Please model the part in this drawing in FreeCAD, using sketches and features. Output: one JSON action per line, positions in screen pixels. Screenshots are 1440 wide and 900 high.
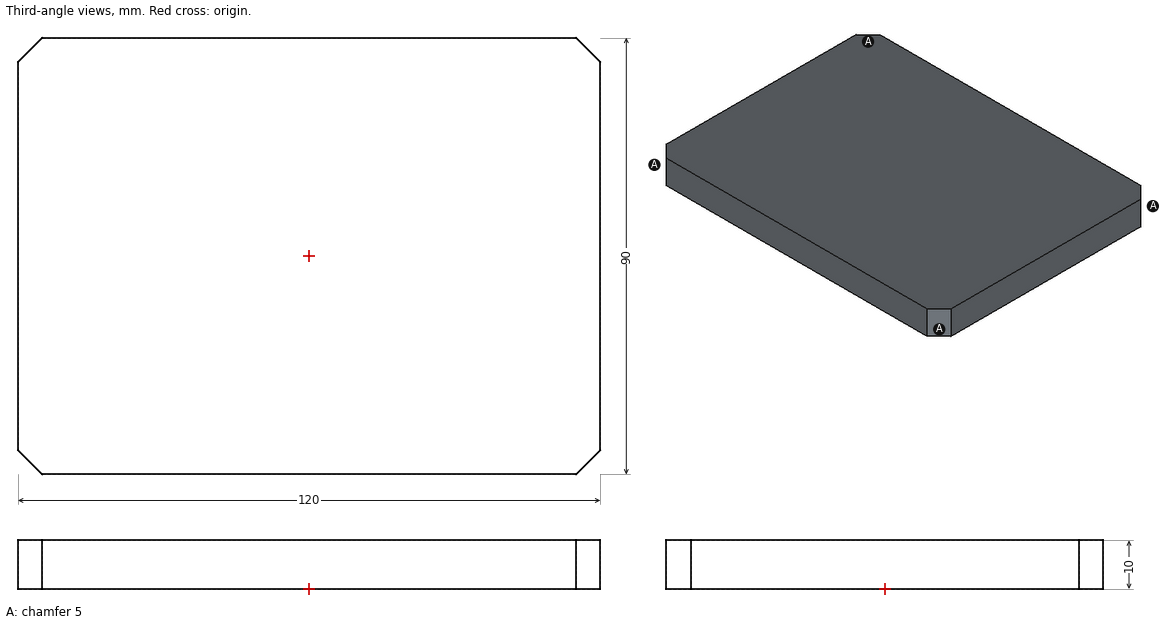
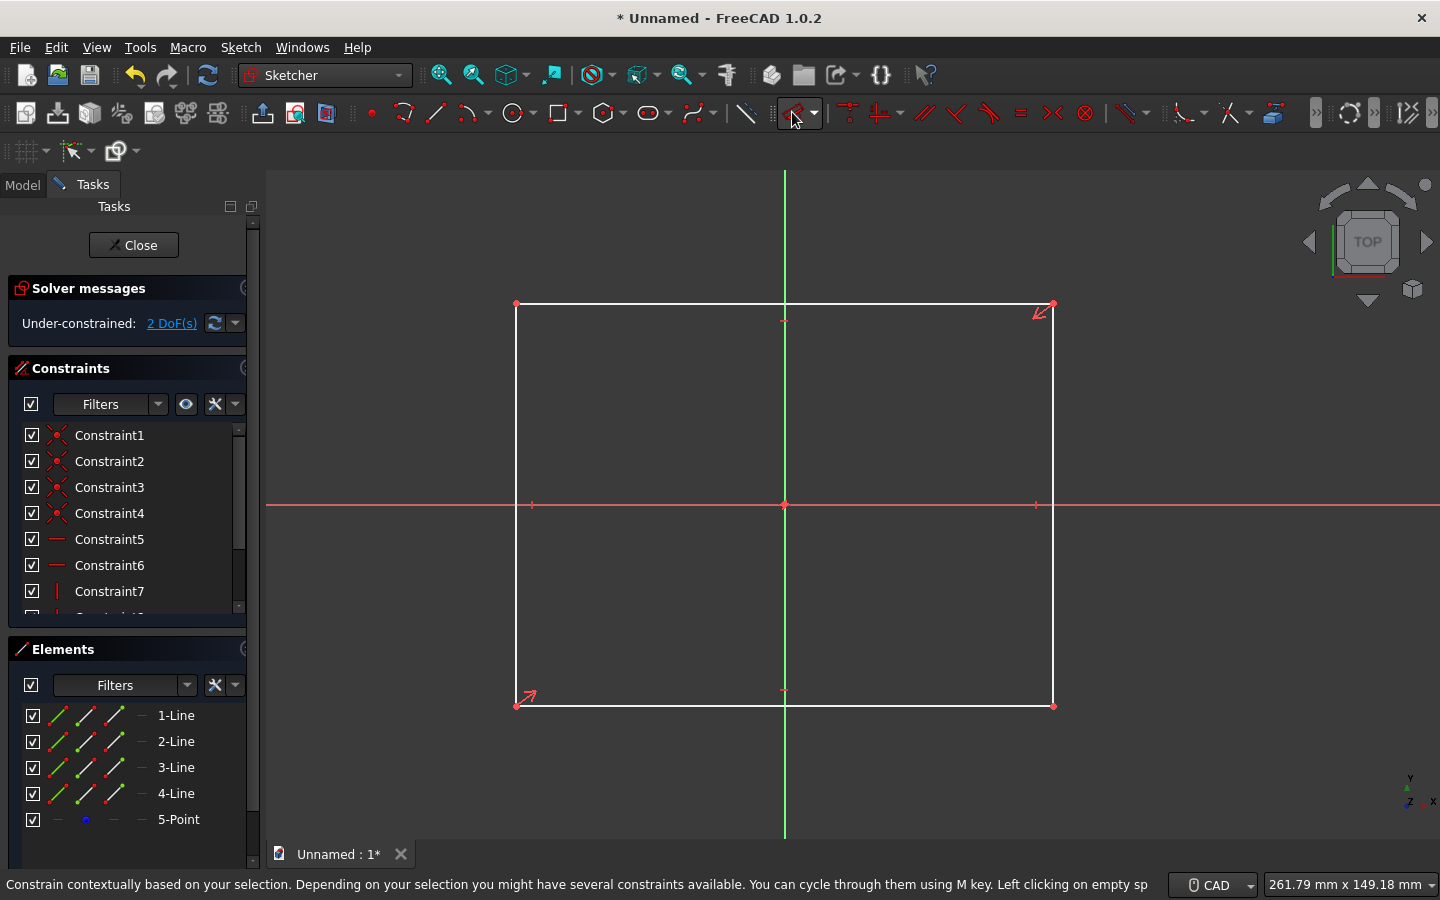
{"action": "left_click", "coordinate": [1053, 585]}
{"action": "left_click", "coordinate": [1087, 412]}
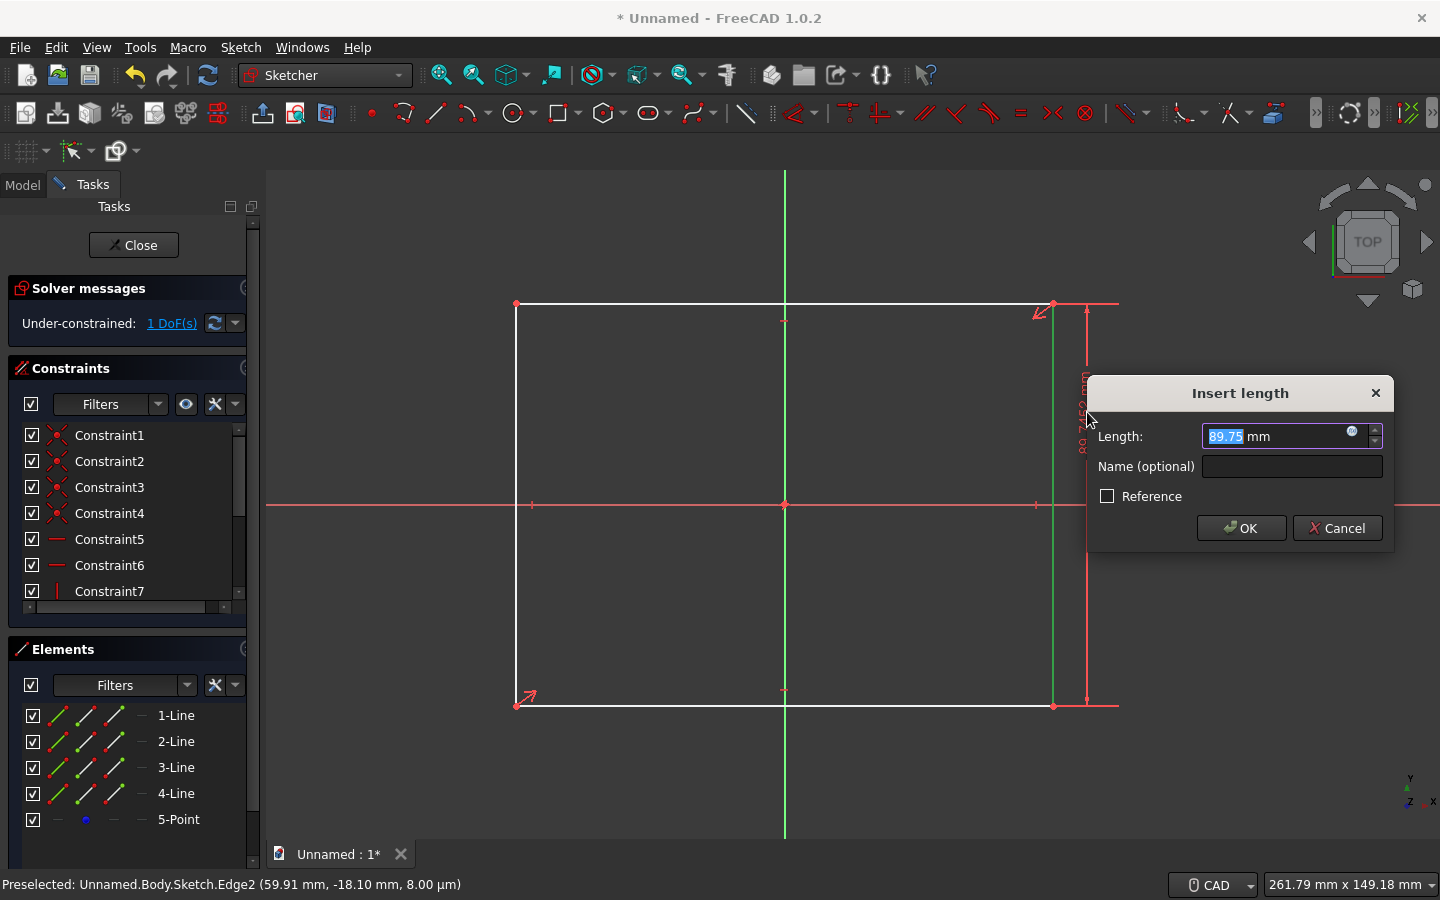
{"action": "type", "text": "90"}
{"action": "key", "text": "Return"}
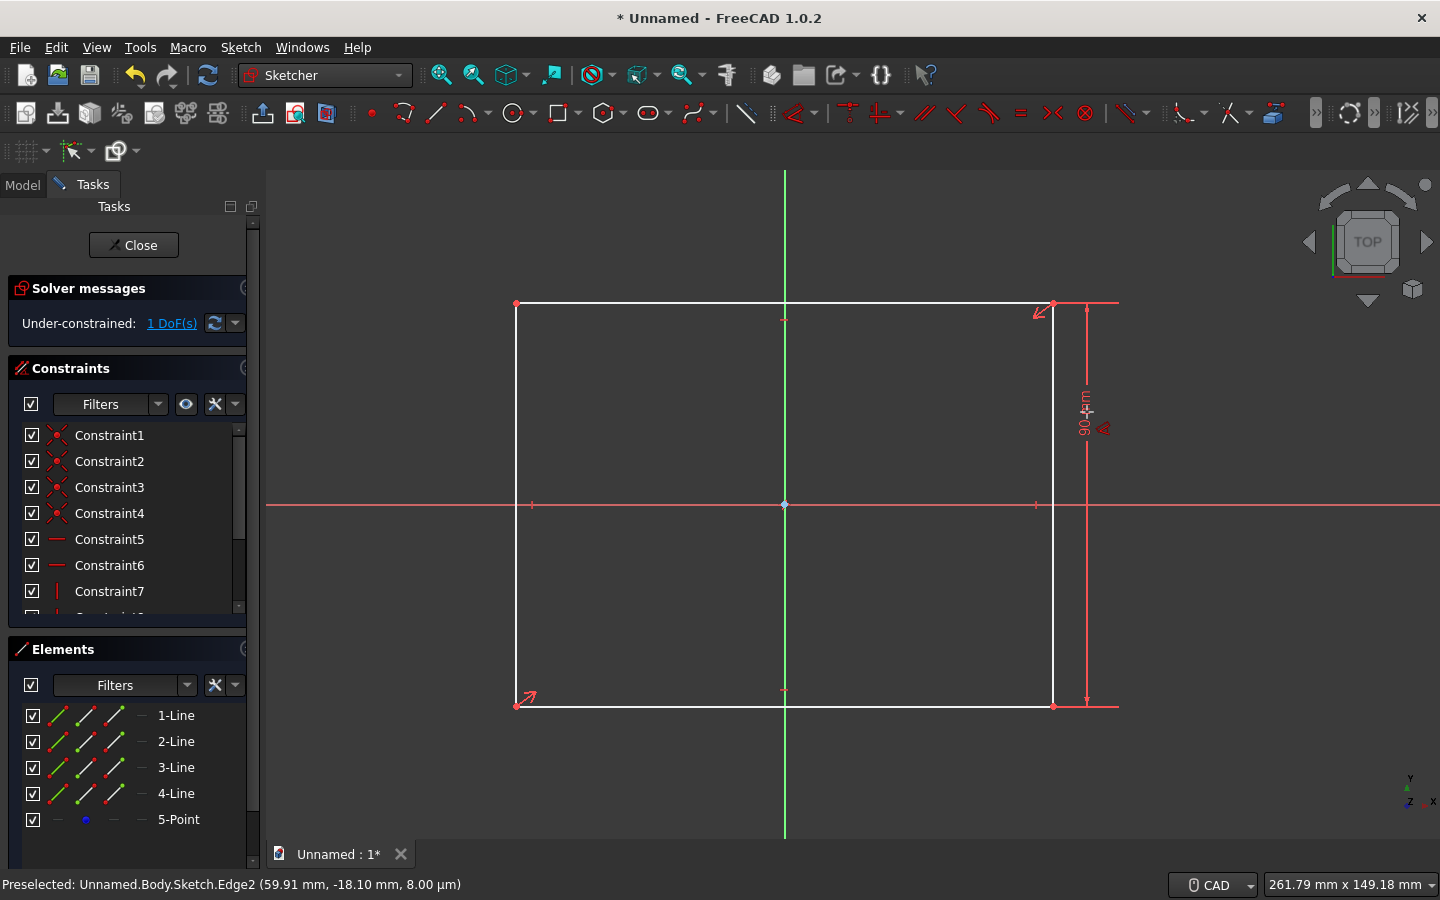
{"action": "left_click", "coordinate": [677, 707]}
{"action": "left_click", "coordinate": [661, 741]}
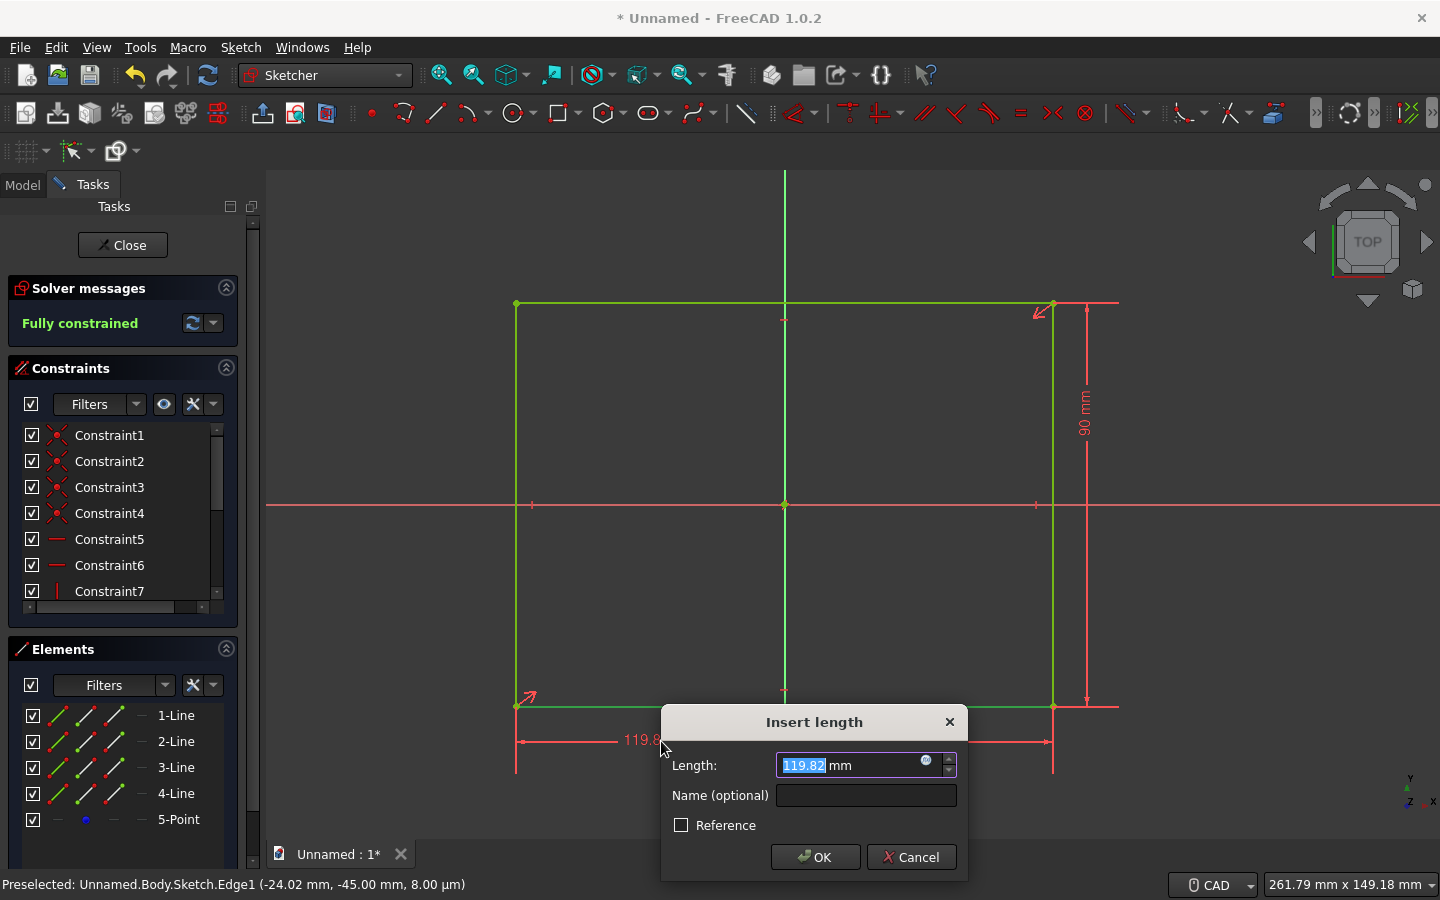
{"action": "type", "text": "120"}
{"action": "key", "text": "Return"}
{"action": "key", "text": "Escape"}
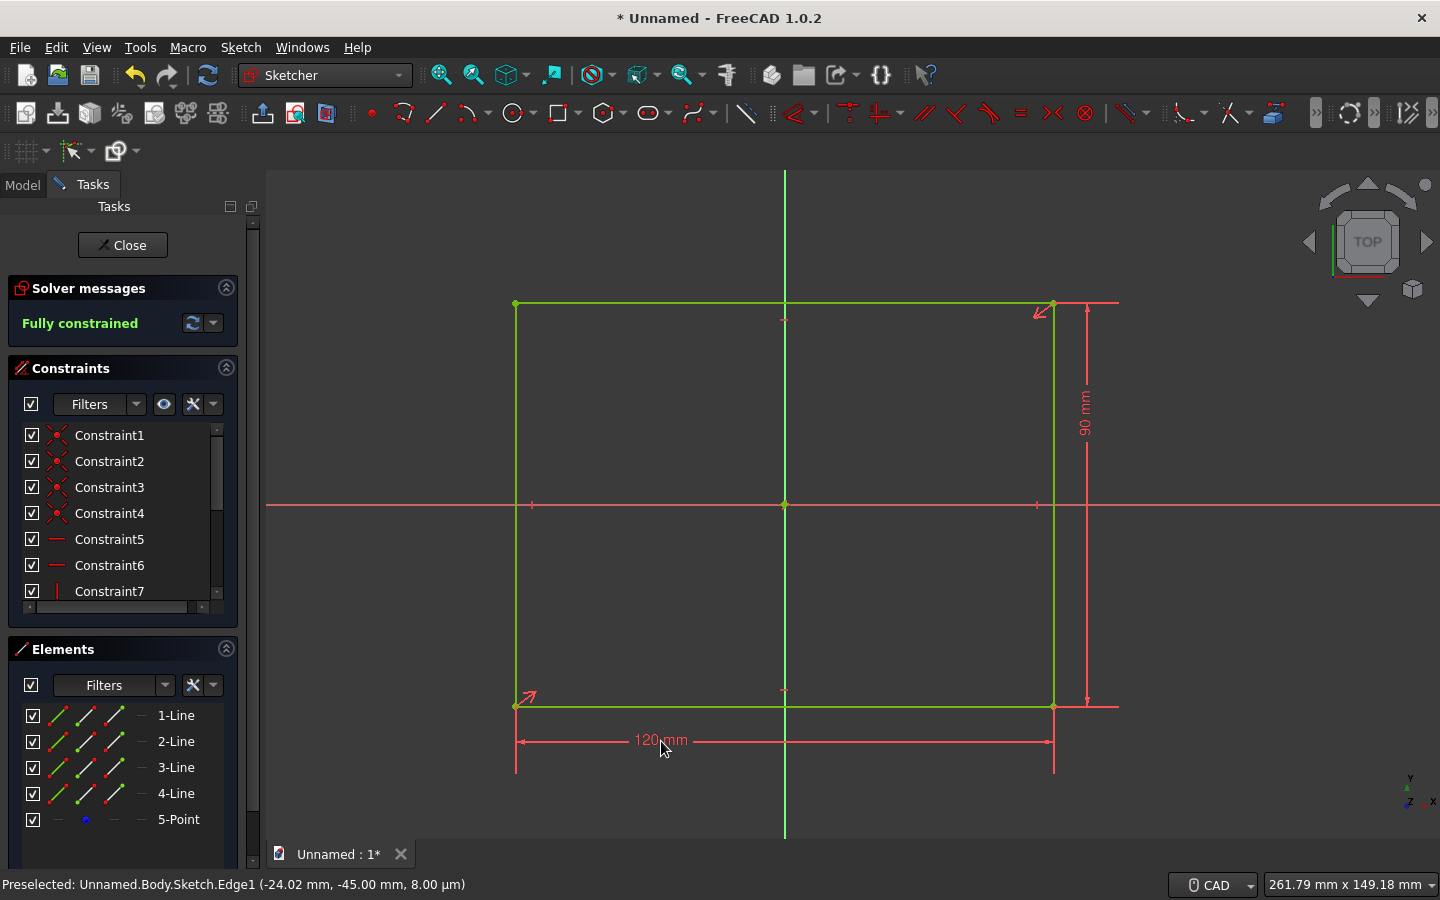
{"action": "left_click", "coordinate": [123, 245]}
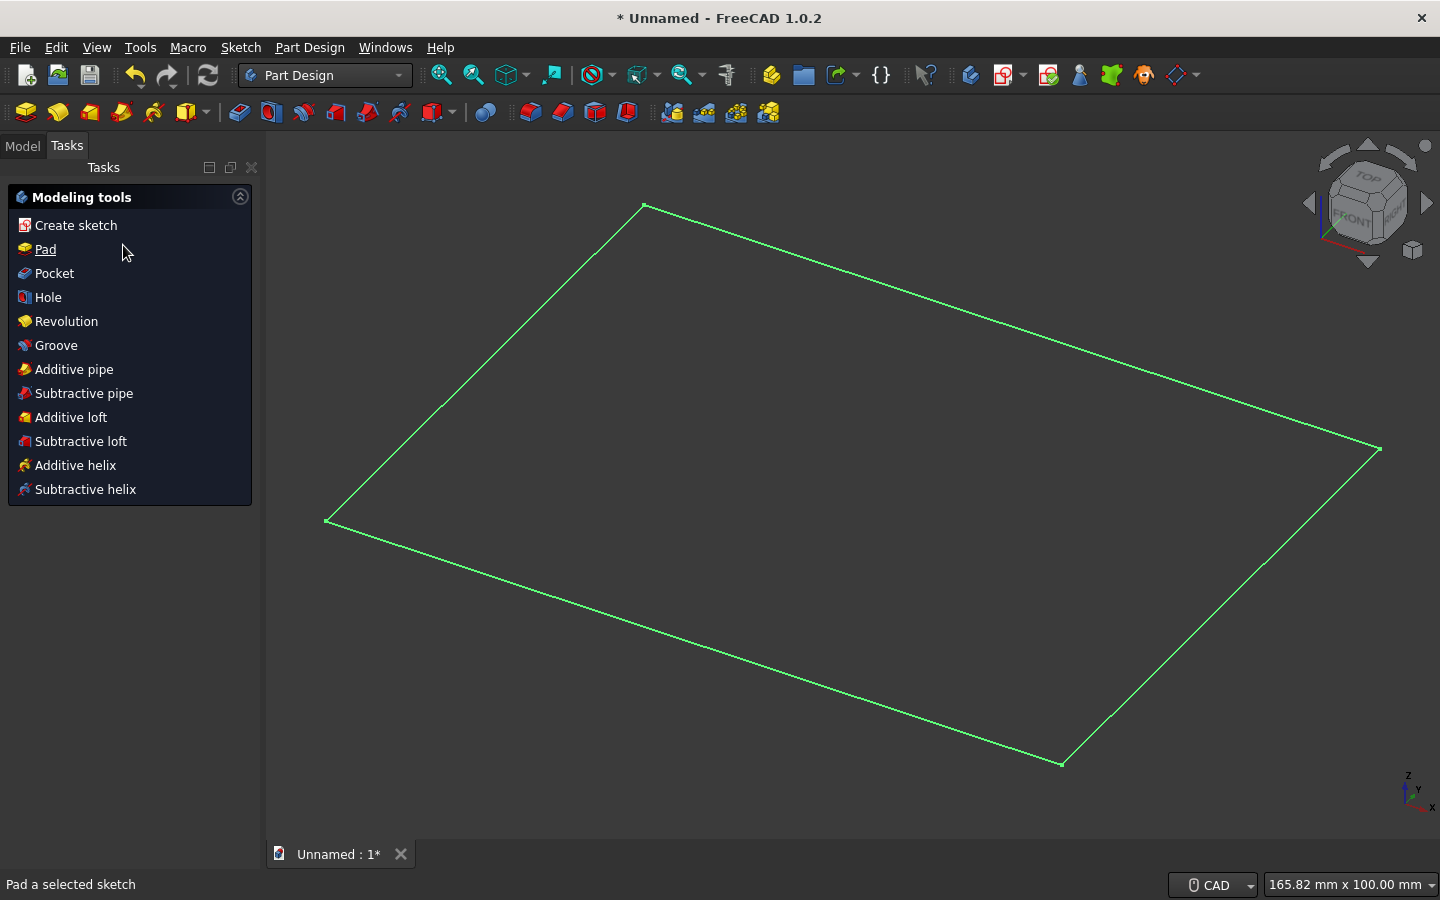
{"action": "left_click", "coordinate": [26, 112]}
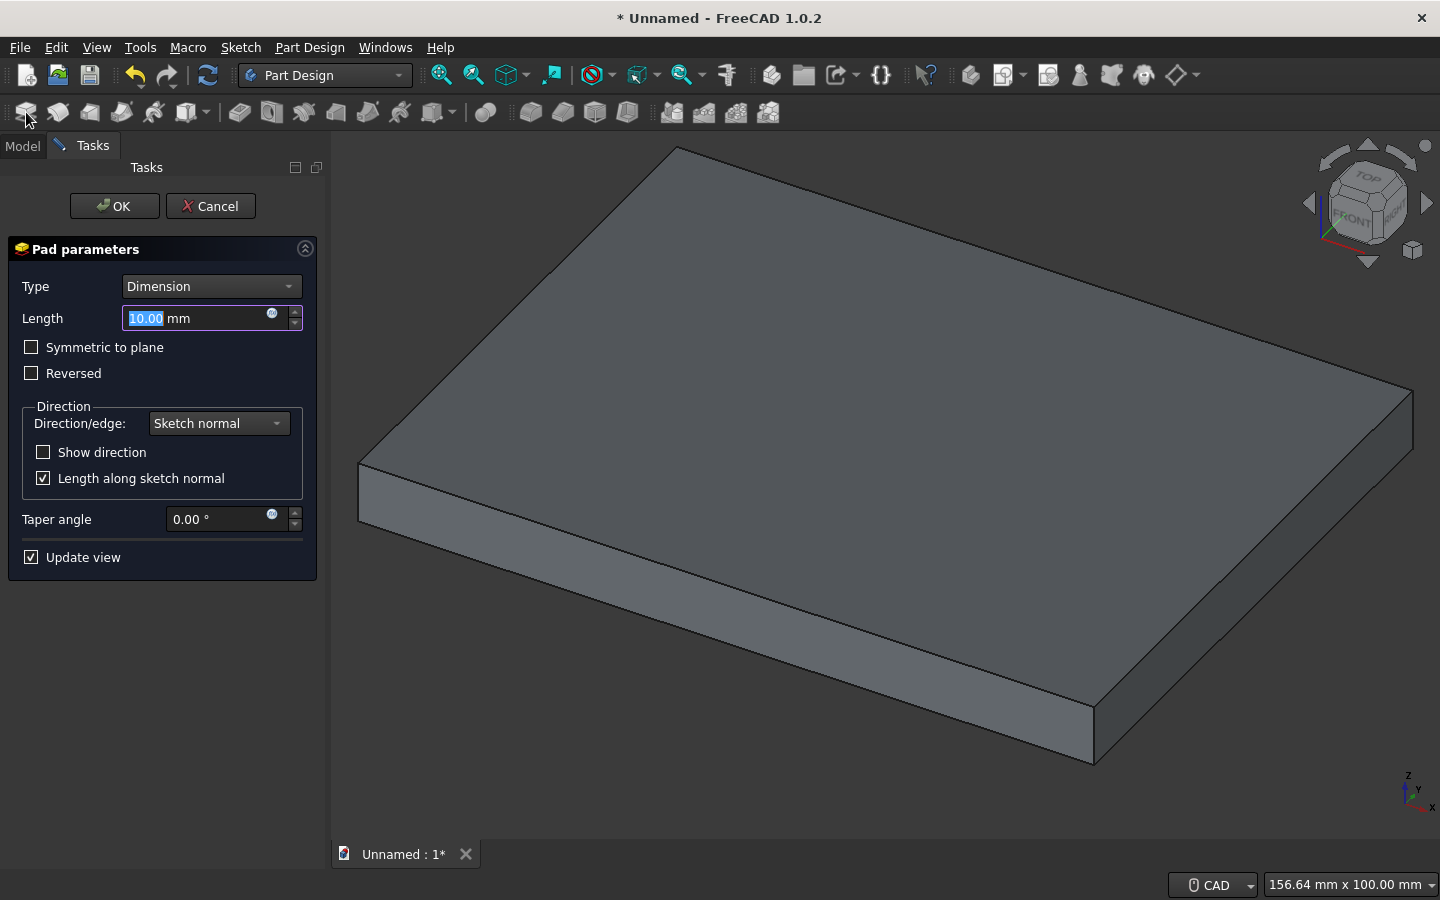
{"action": "type", "text": "10"}
{"action": "key", "text": "Tab"}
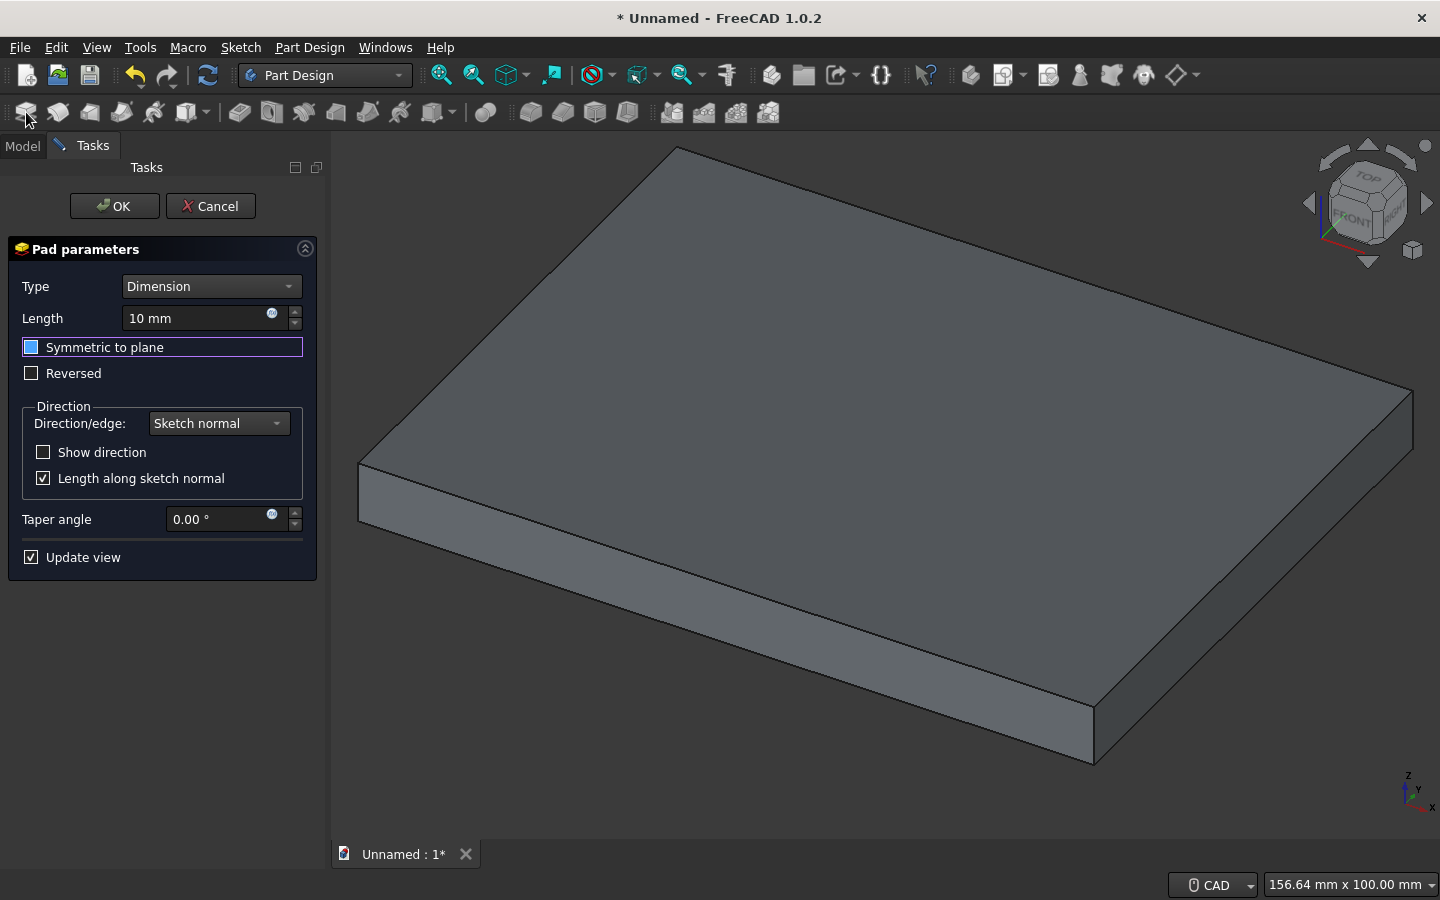
{"action": "left_click", "coordinate": [115, 206]}